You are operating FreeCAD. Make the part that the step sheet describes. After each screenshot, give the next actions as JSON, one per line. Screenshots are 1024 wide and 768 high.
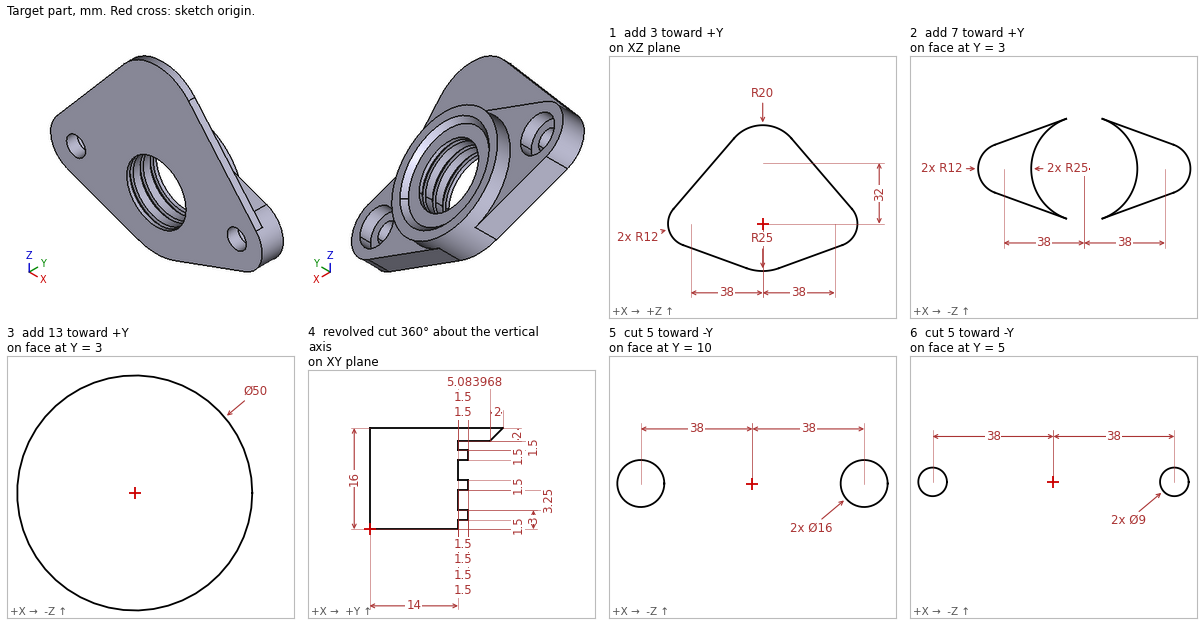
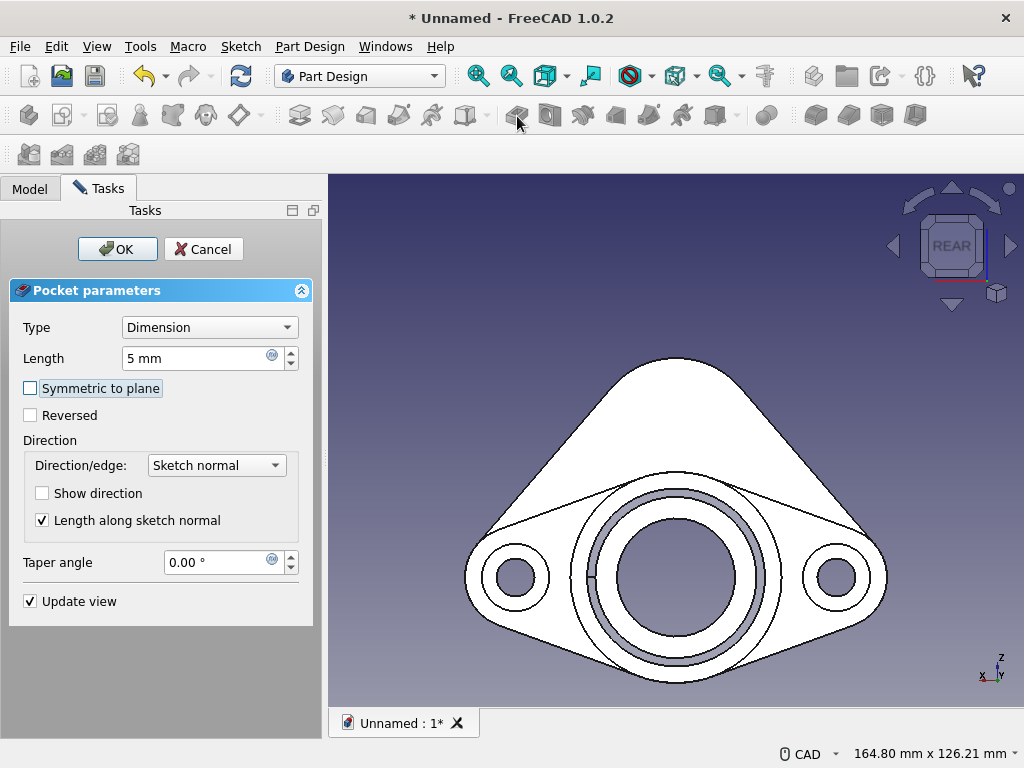
{"action": "left_click", "coordinate": [118, 249]}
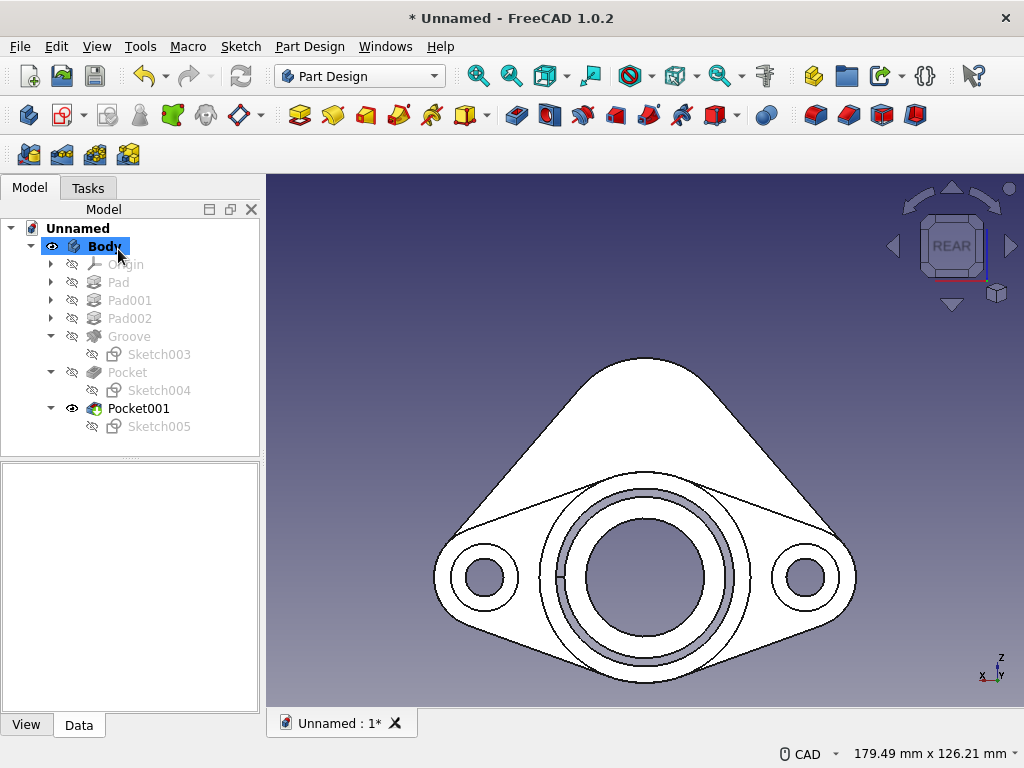
{"action": "key", "text": "0"}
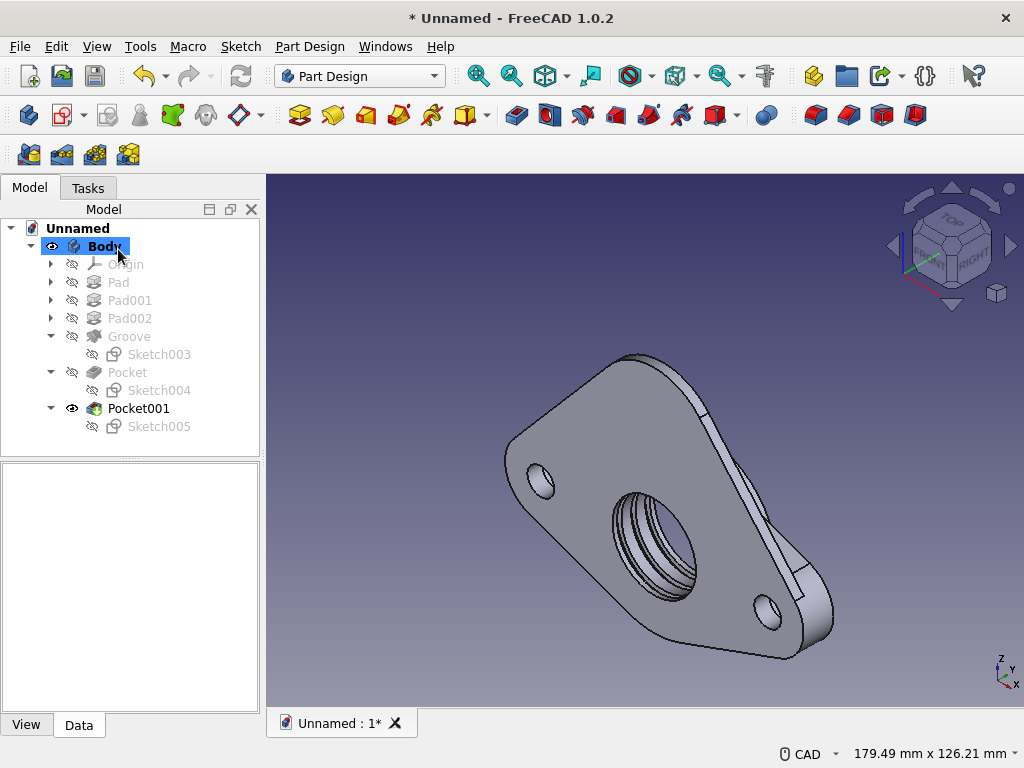
{"action": "left_click", "coordinate": [479, 76]}